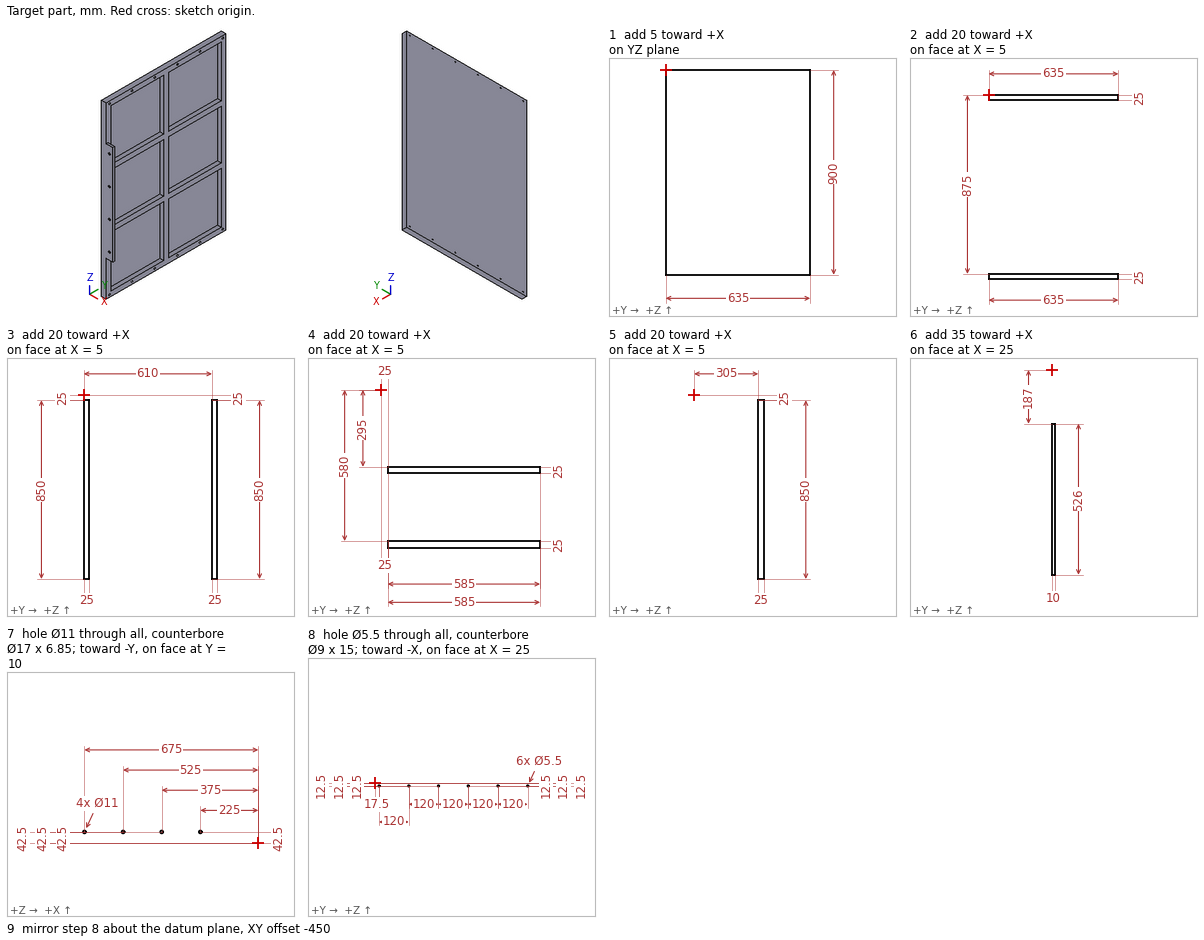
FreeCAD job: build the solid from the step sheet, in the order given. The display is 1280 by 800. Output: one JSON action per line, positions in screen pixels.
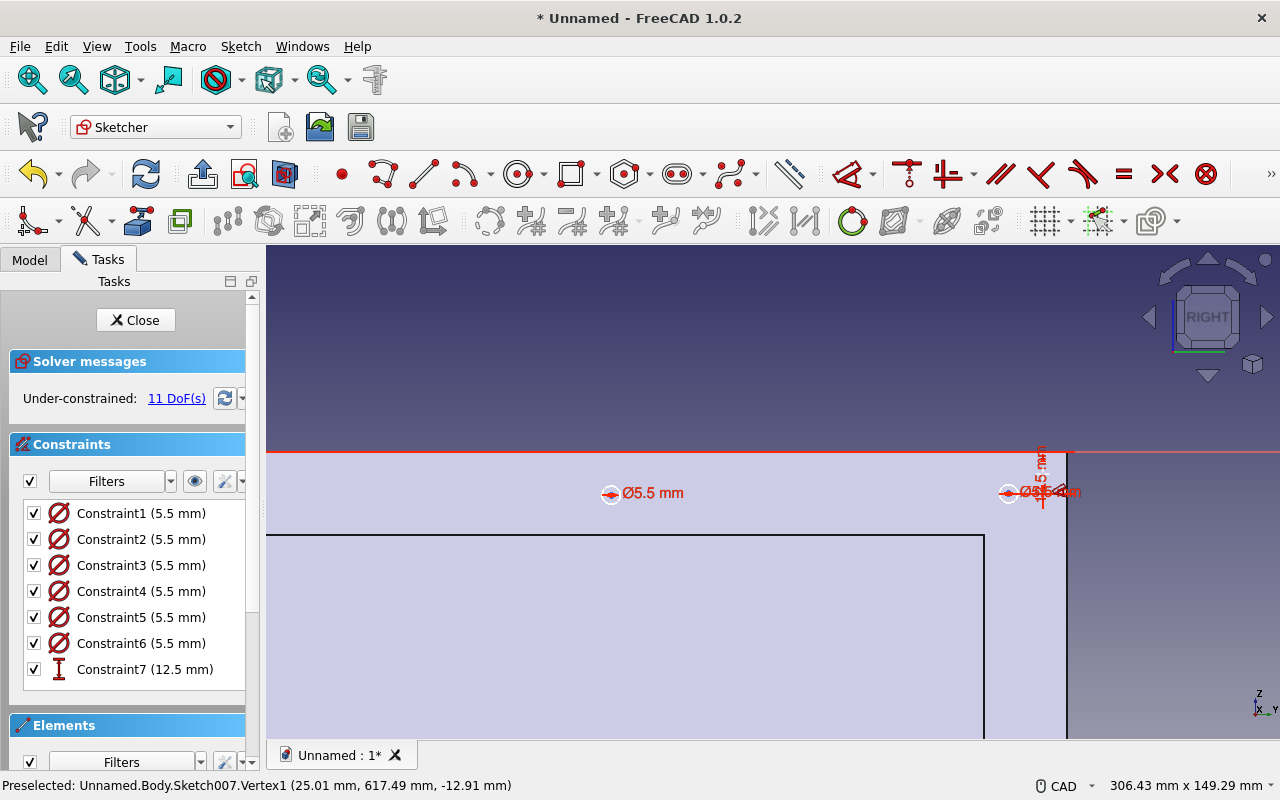
{"action": "left_click", "coordinate": [611, 495]}
{"action": "left_click", "coordinate": [645, 474]}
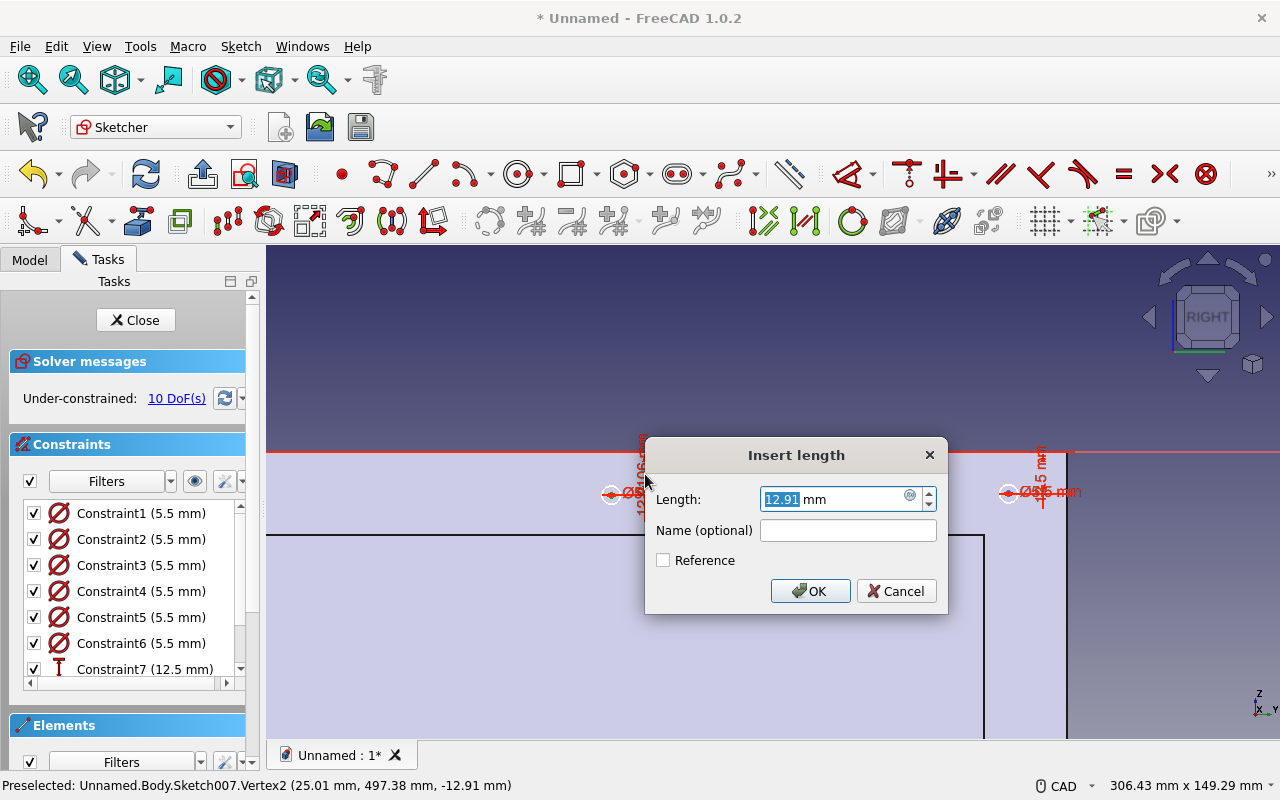
{"action": "type", "text": "12.5"}
{"action": "key", "text": "Return"}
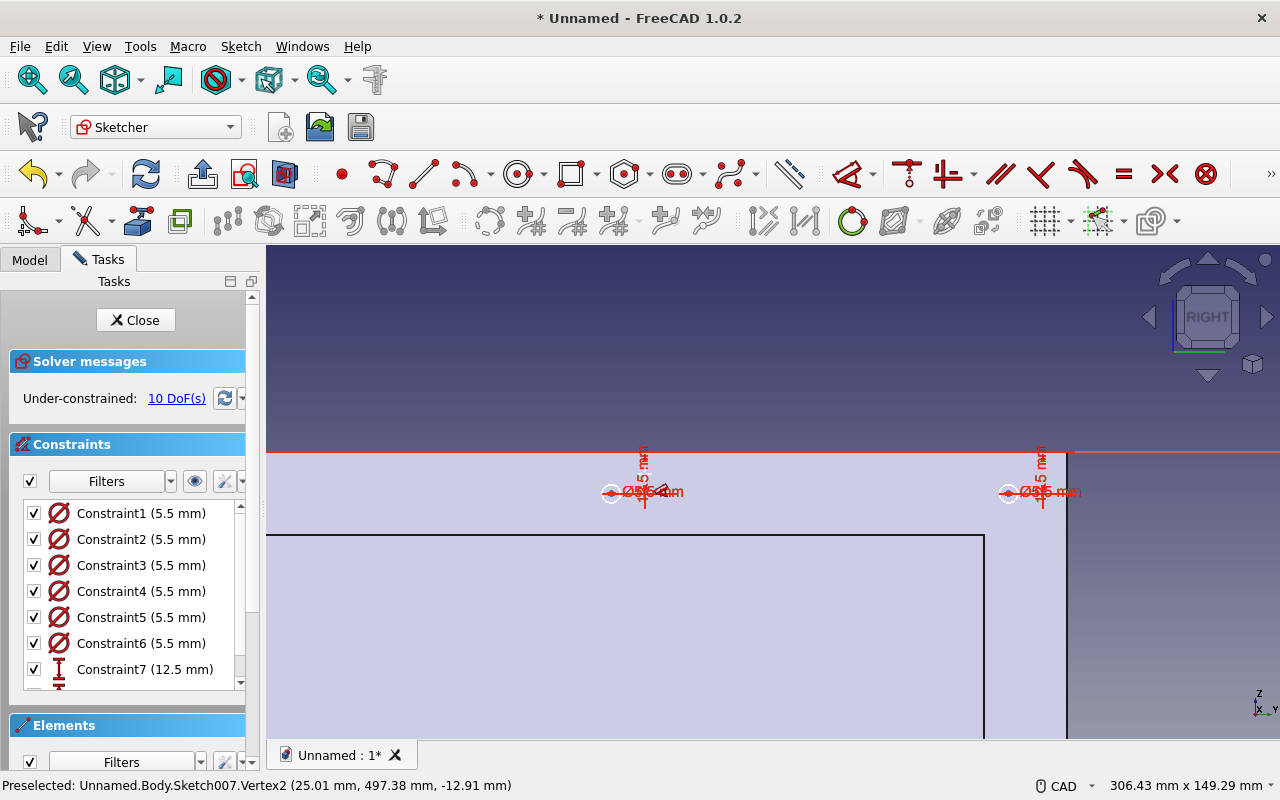
{"action": "scroll", "coordinate": [1012, 498], "scroll_direction": "down", "scroll_amount": 6}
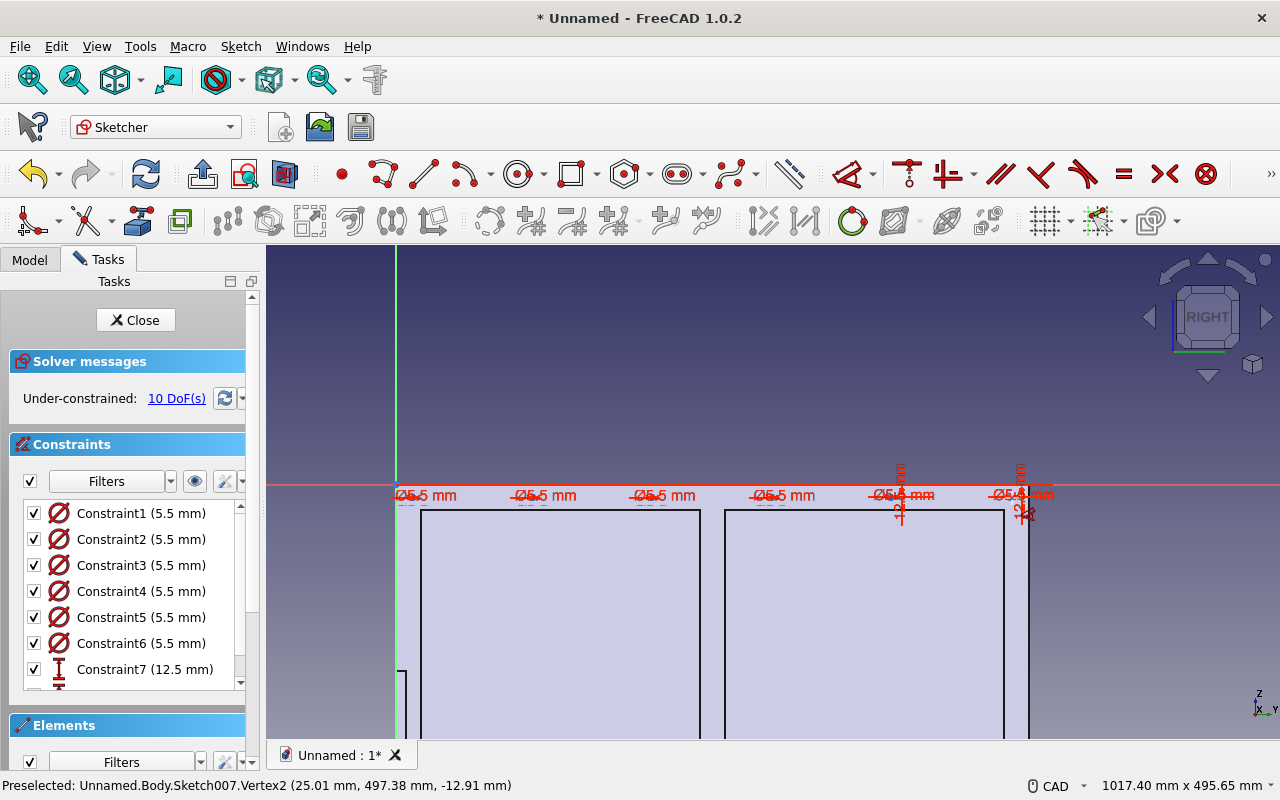
{"action": "scroll", "coordinate": [772, 498], "scroll_direction": "up", "scroll_amount": 6}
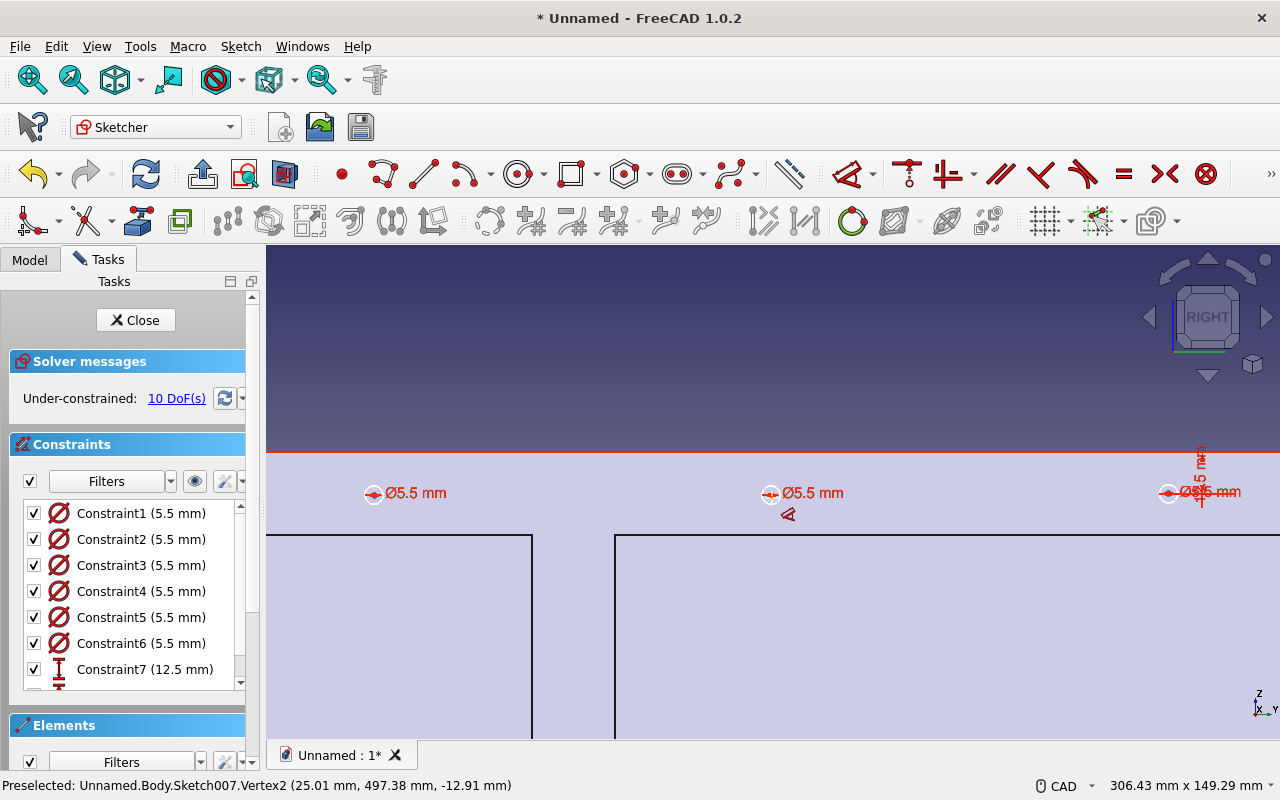
{"action": "left_click", "coordinate": [771, 495]}
{"action": "left_click", "coordinate": [805, 474]}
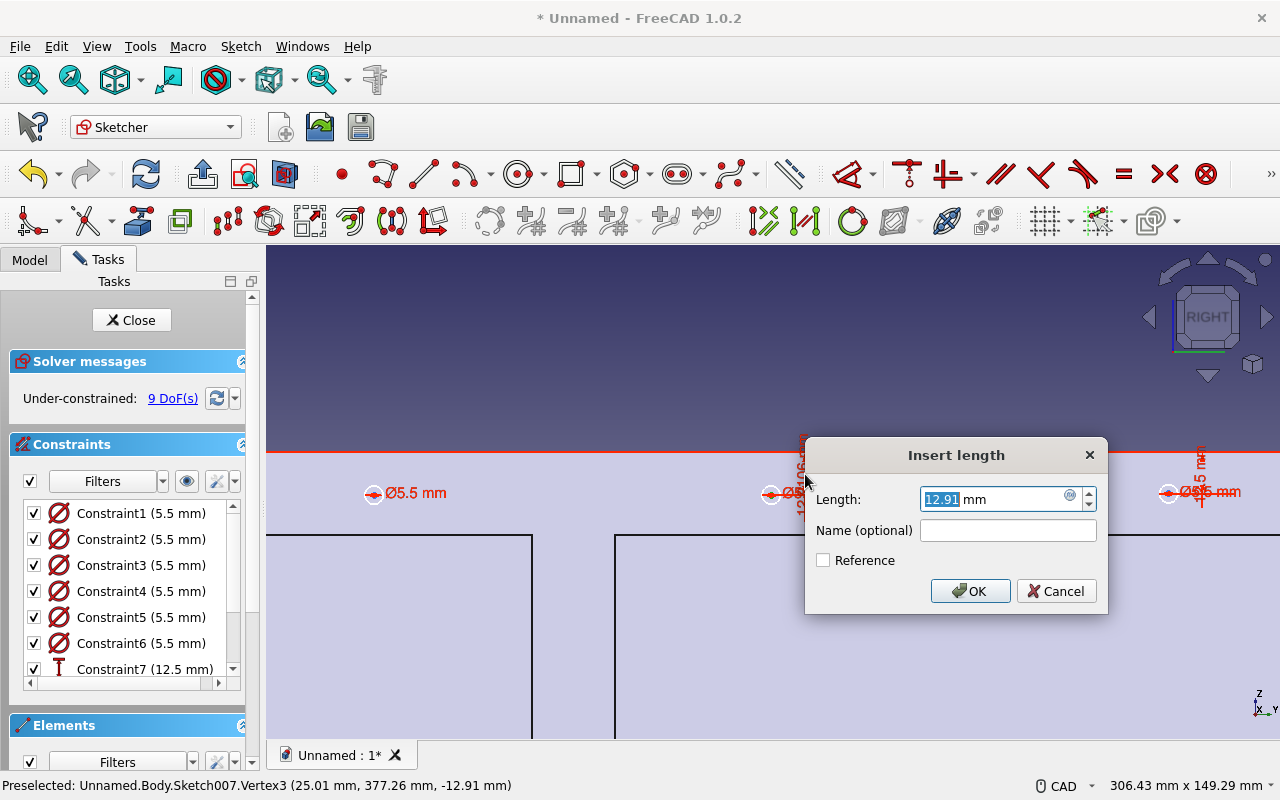
{"action": "type", "text": "12.5"}
{"action": "key", "text": "Return"}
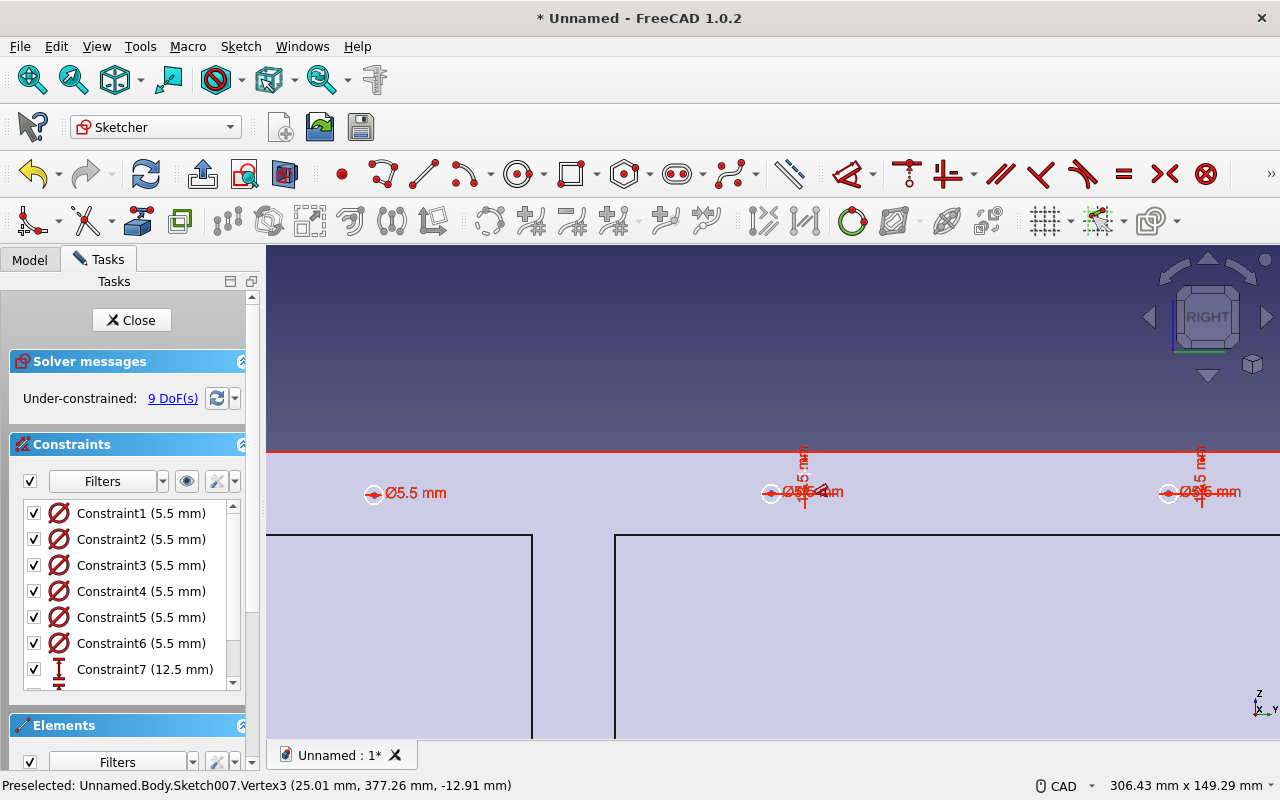
{"action": "left_click", "coordinate": [374, 495]}
{"action": "left_click", "coordinate": [408, 474]}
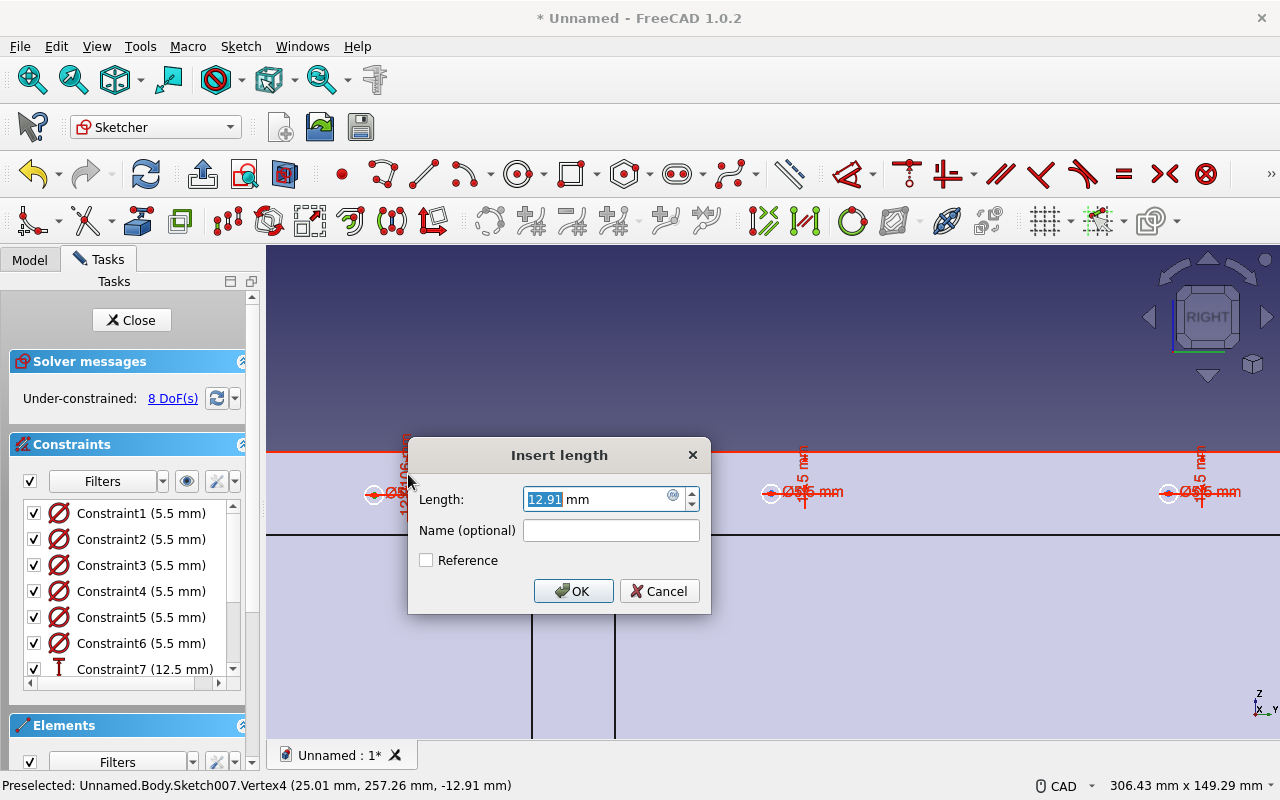
{"action": "type", "text": "12.5"}
{"action": "key", "text": "Return"}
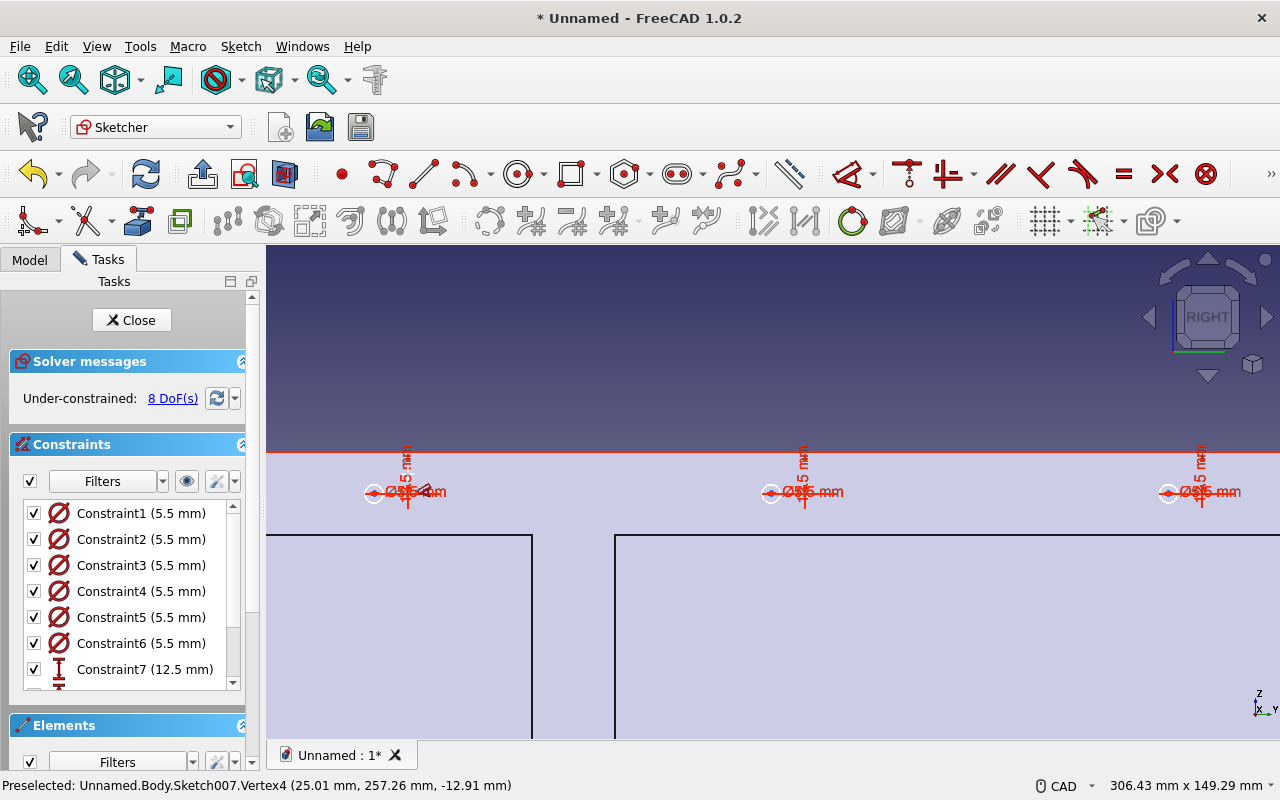
{"action": "scroll", "coordinate": [772, 498], "scroll_direction": "down", "scroll_amount": 6}